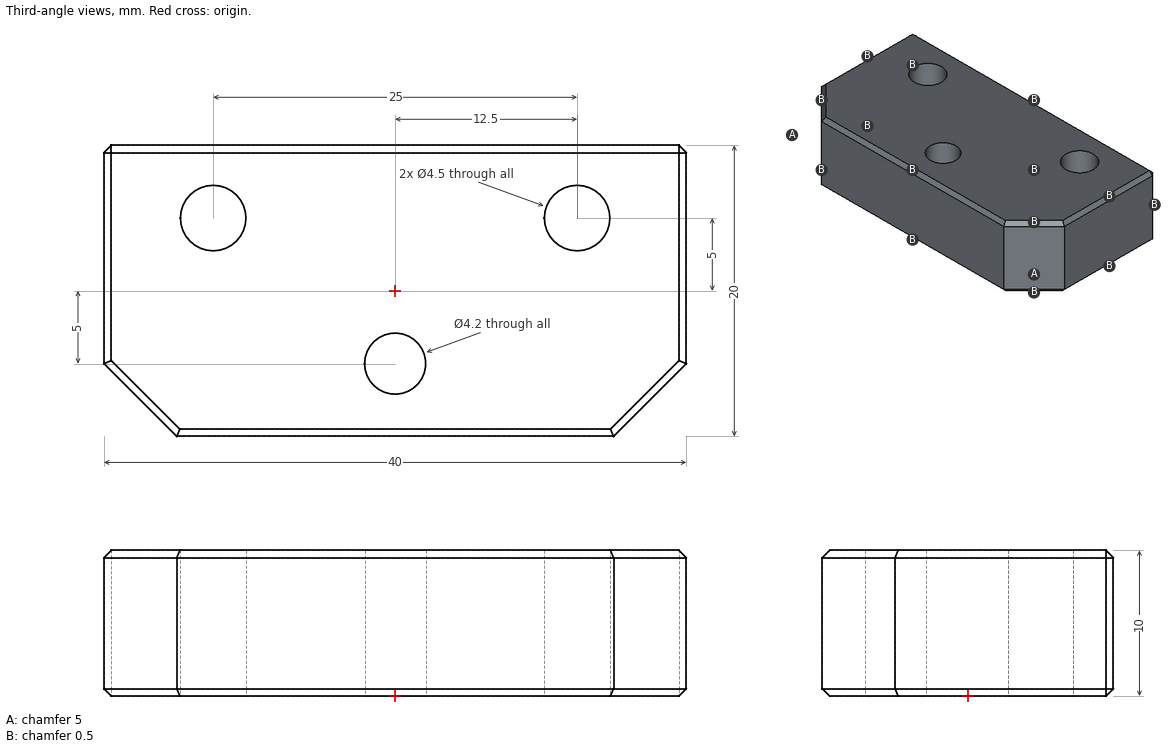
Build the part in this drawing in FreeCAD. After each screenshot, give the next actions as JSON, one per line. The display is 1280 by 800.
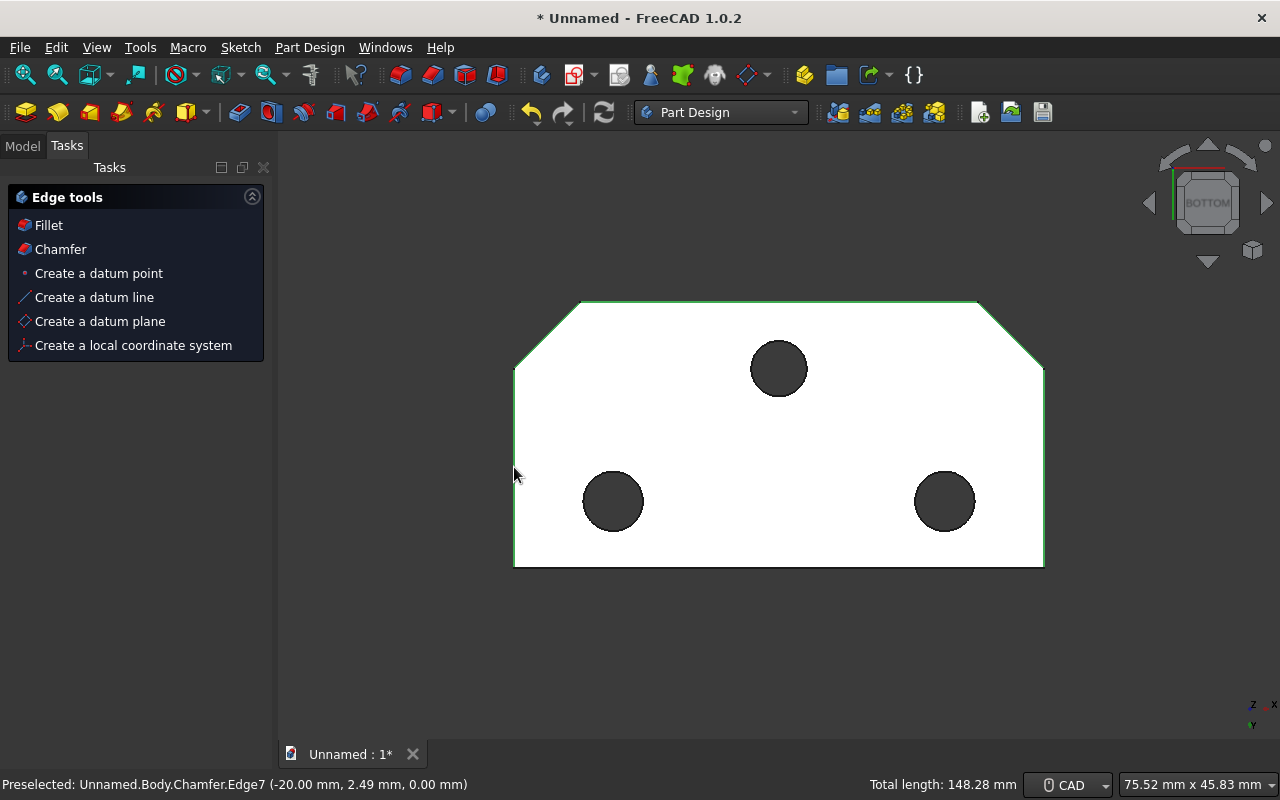
{"action": "key", "text": "4"}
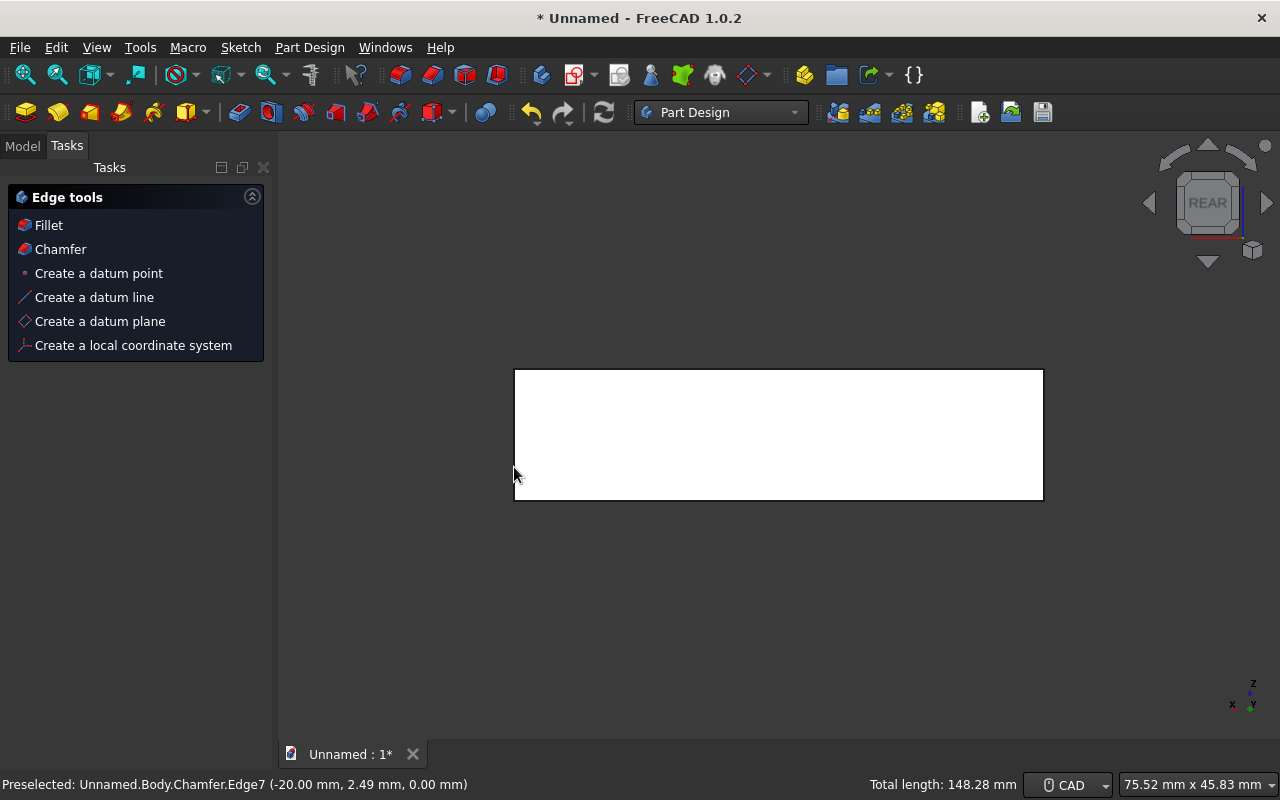
{"action": "left_click", "coordinate": [627, 434], "text": "ctrl"}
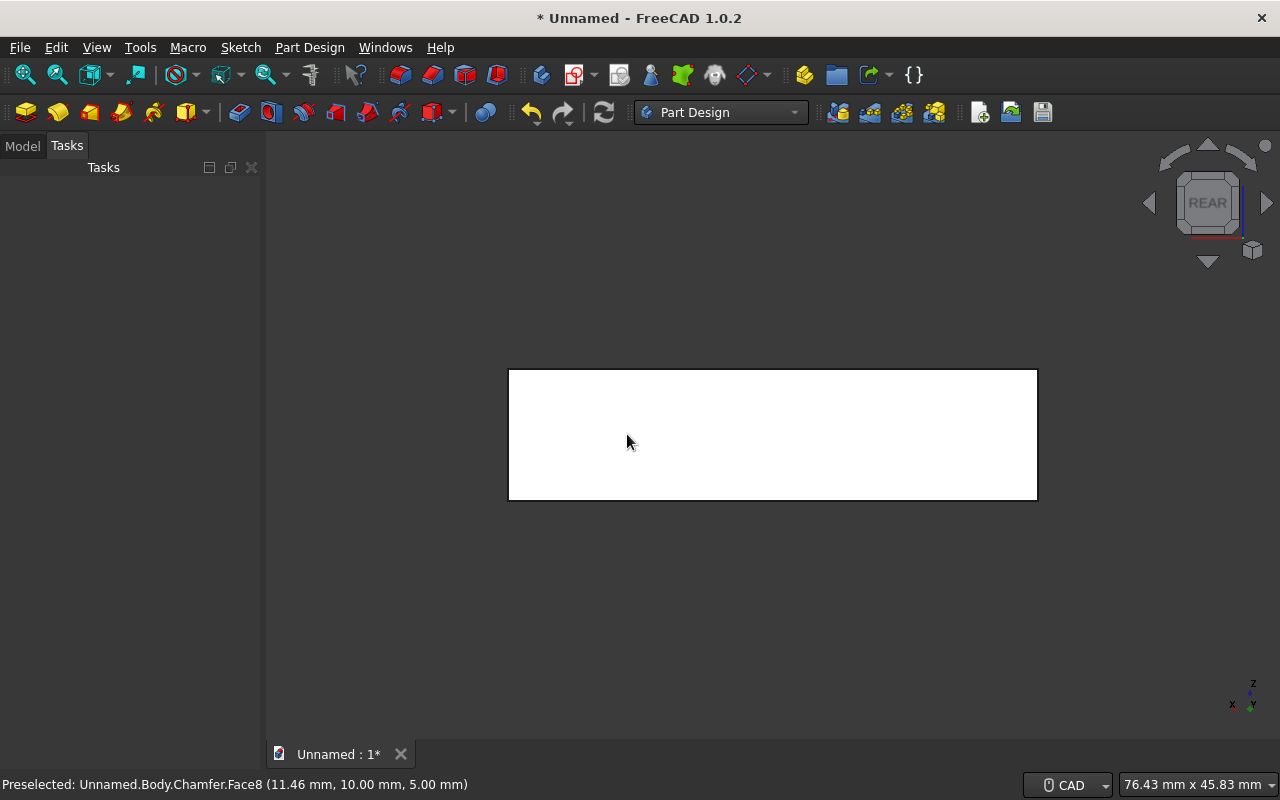
{"action": "left_click", "coordinate": [434, 76]}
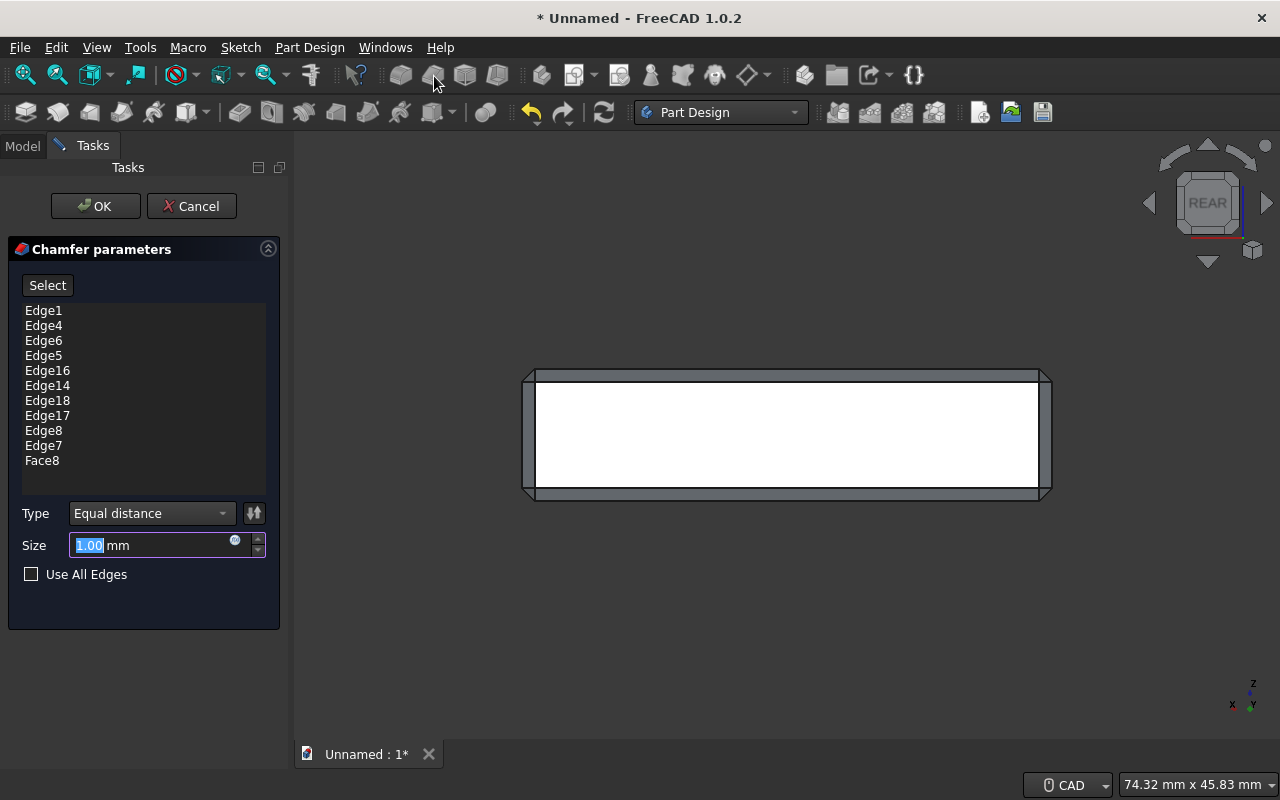
{"action": "type", "text": "0.5"}
{"action": "key", "text": "Tab"}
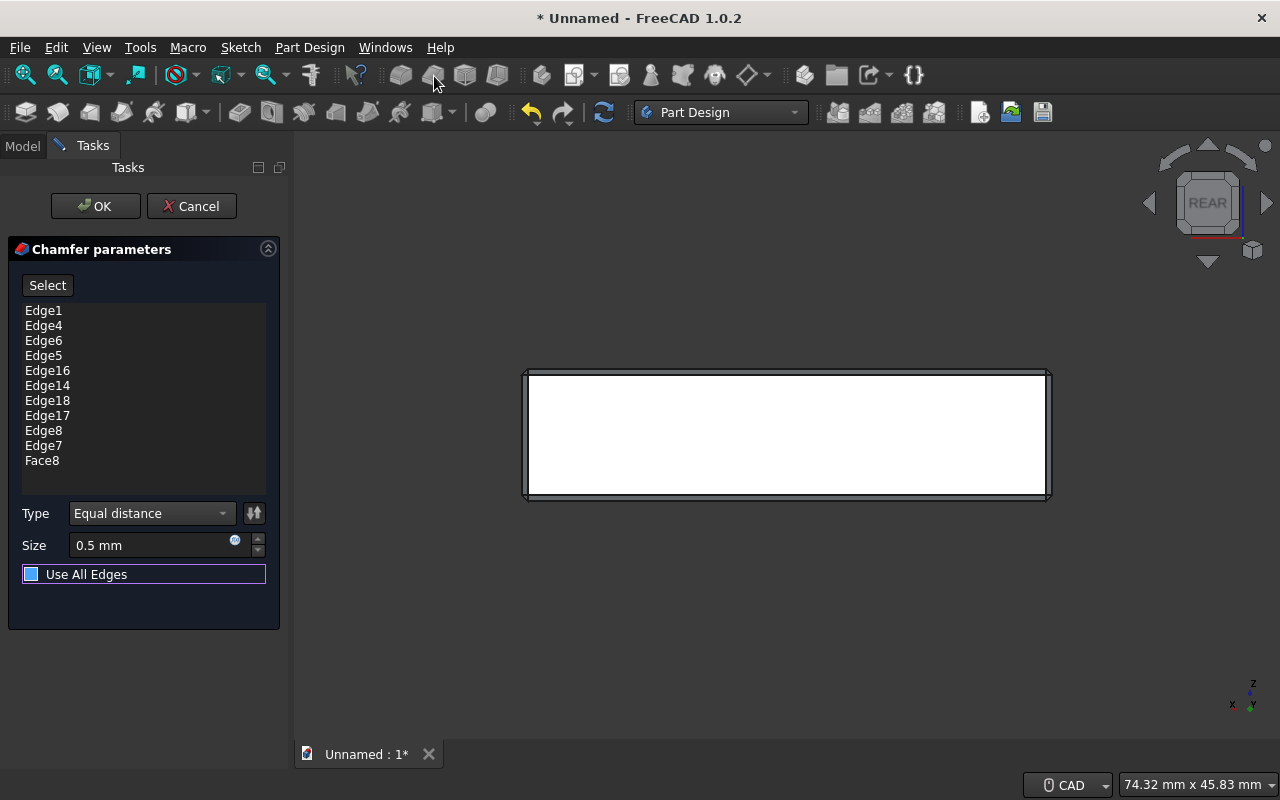
{"action": "left_click", "coordinate": [96, 206]}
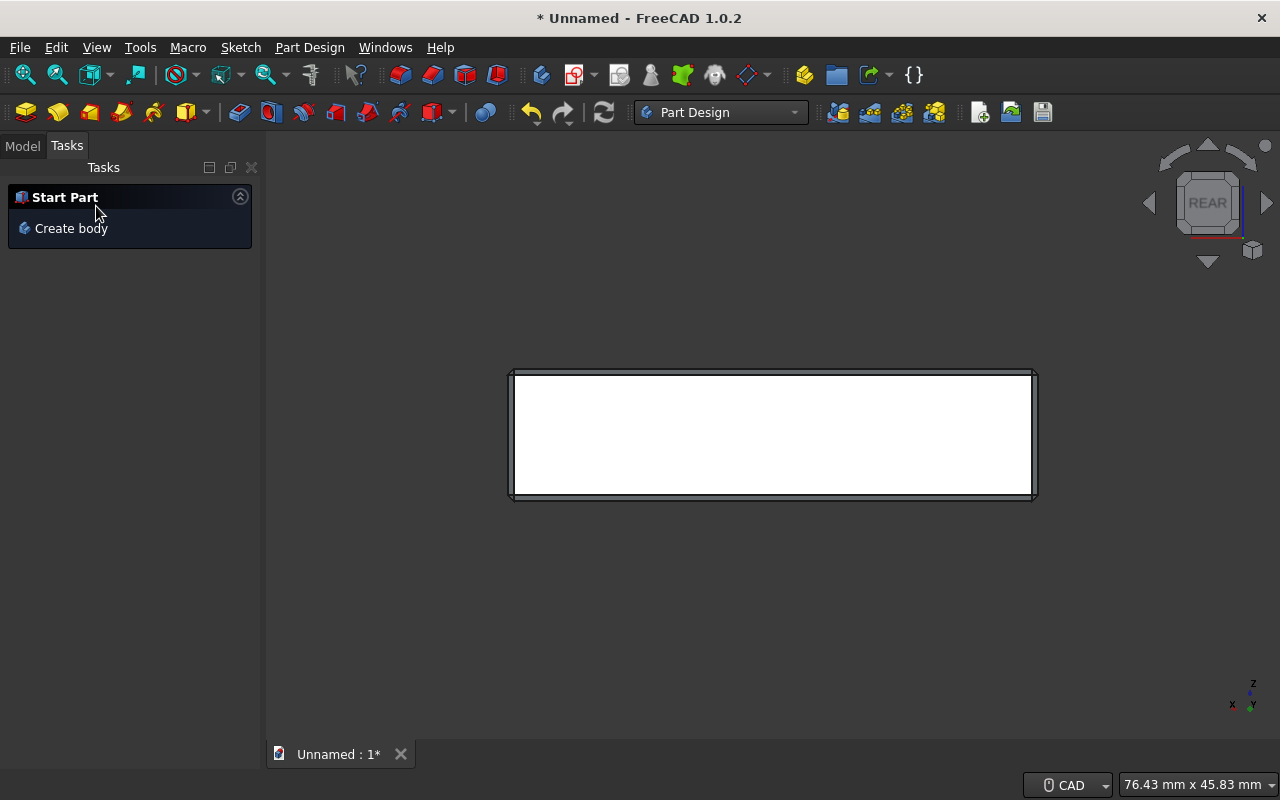
{"action": "key", "text": "0"}